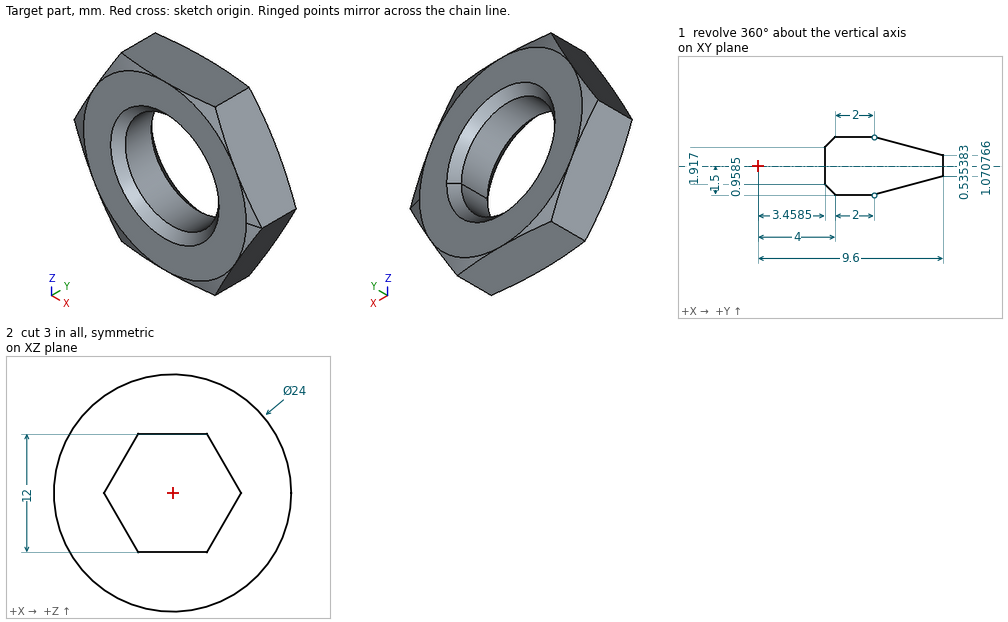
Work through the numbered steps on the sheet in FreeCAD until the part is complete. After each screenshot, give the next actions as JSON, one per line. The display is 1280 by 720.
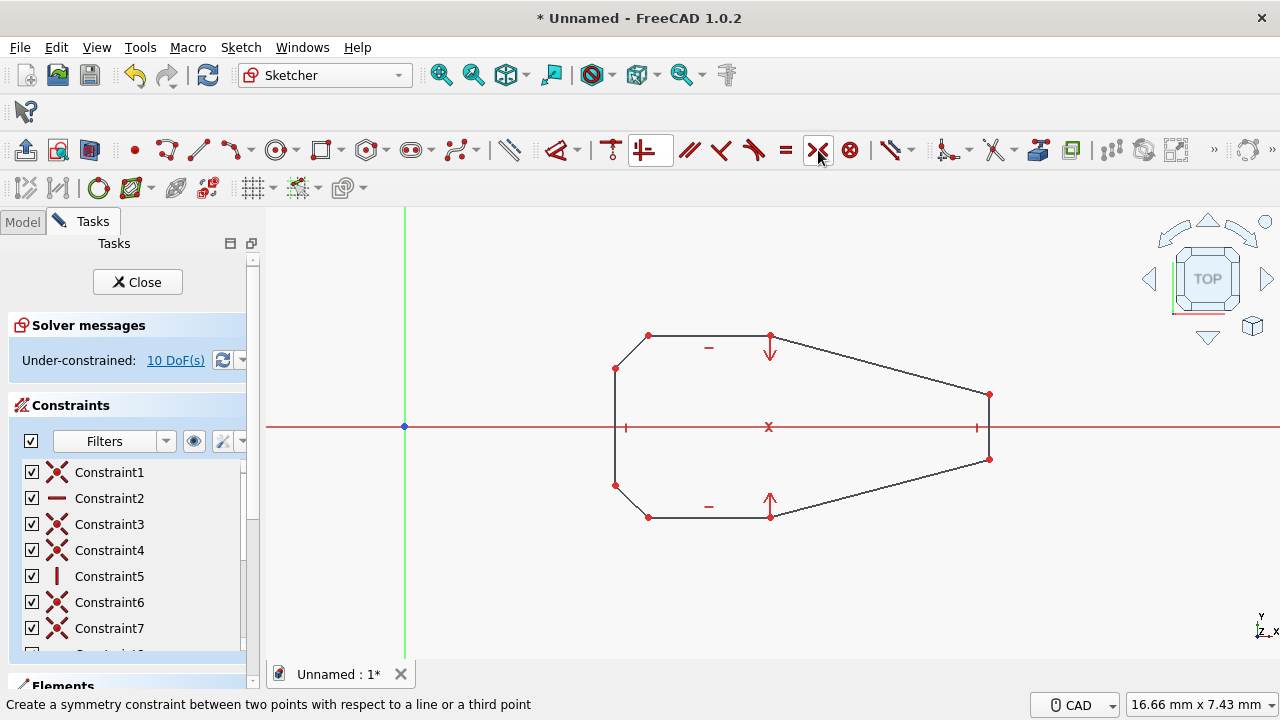
{"action": "left_click", "coordinate": [556, 150]}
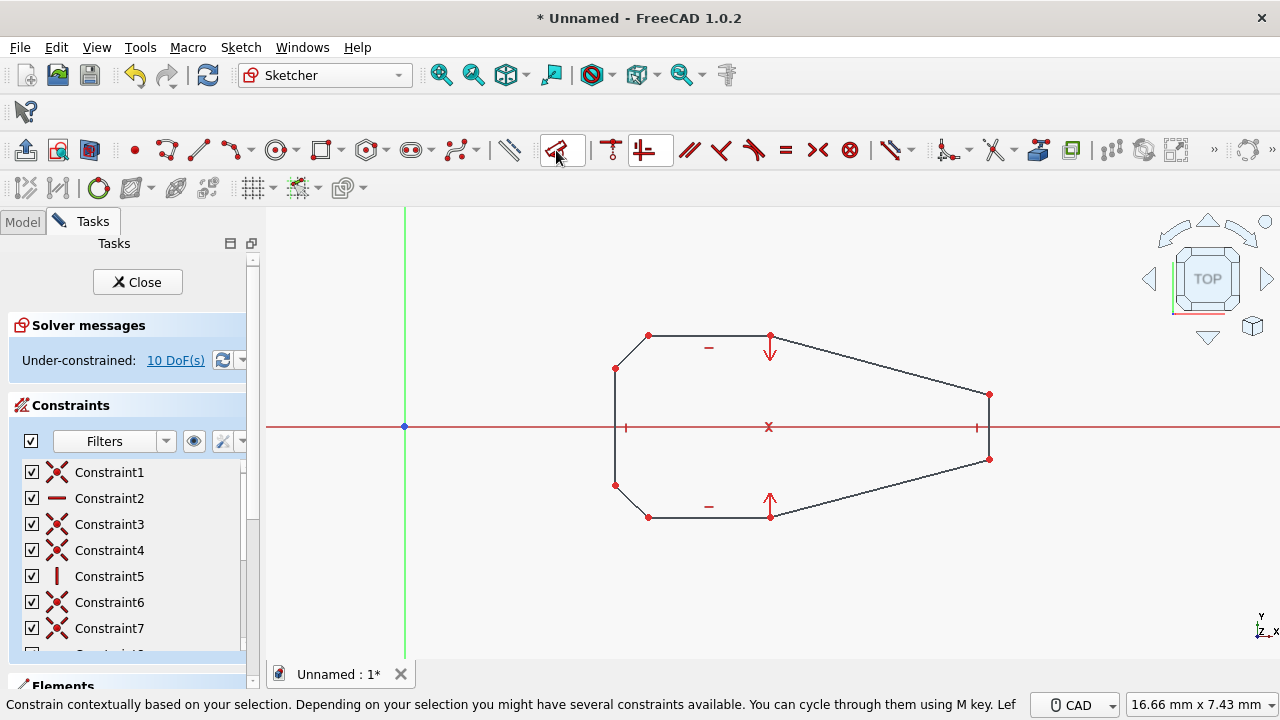
{"action": "left_click", "coordinate": [685, 518]}
{"action": "left_click", "coordinate": [709, 552]}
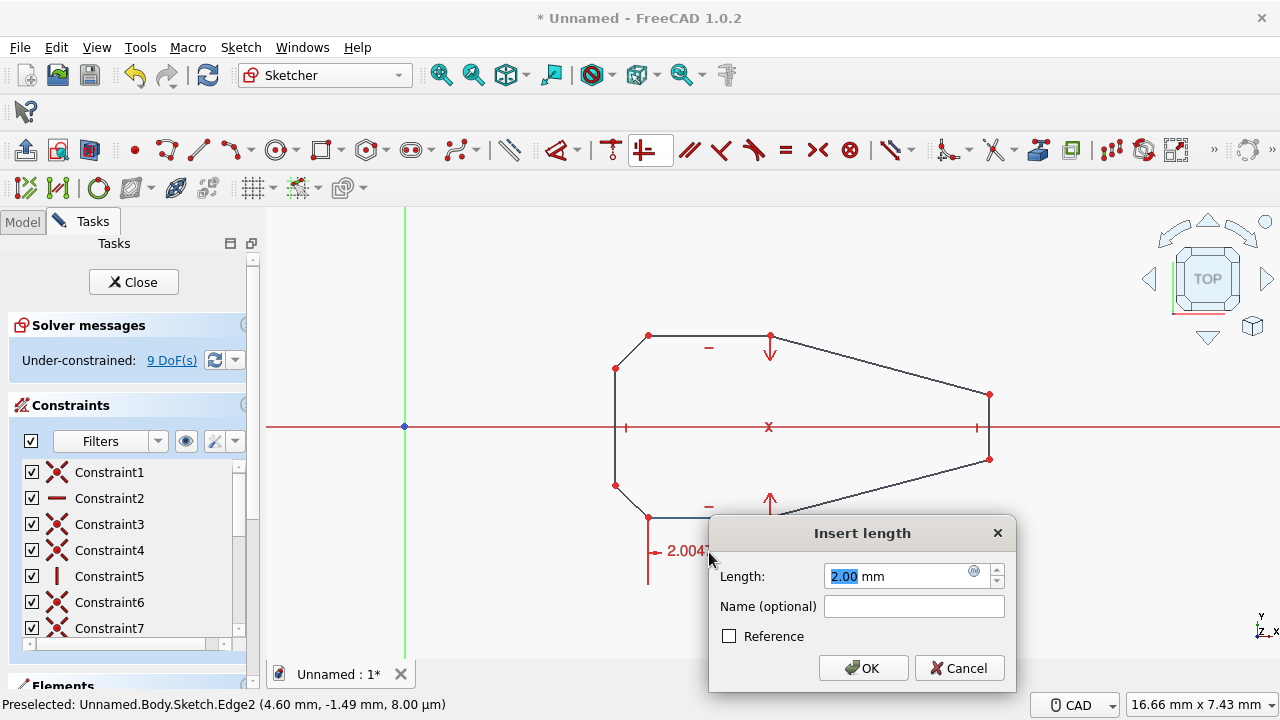
{"action": "type", "text": "2"}
{"action": "key", "text": "Return"}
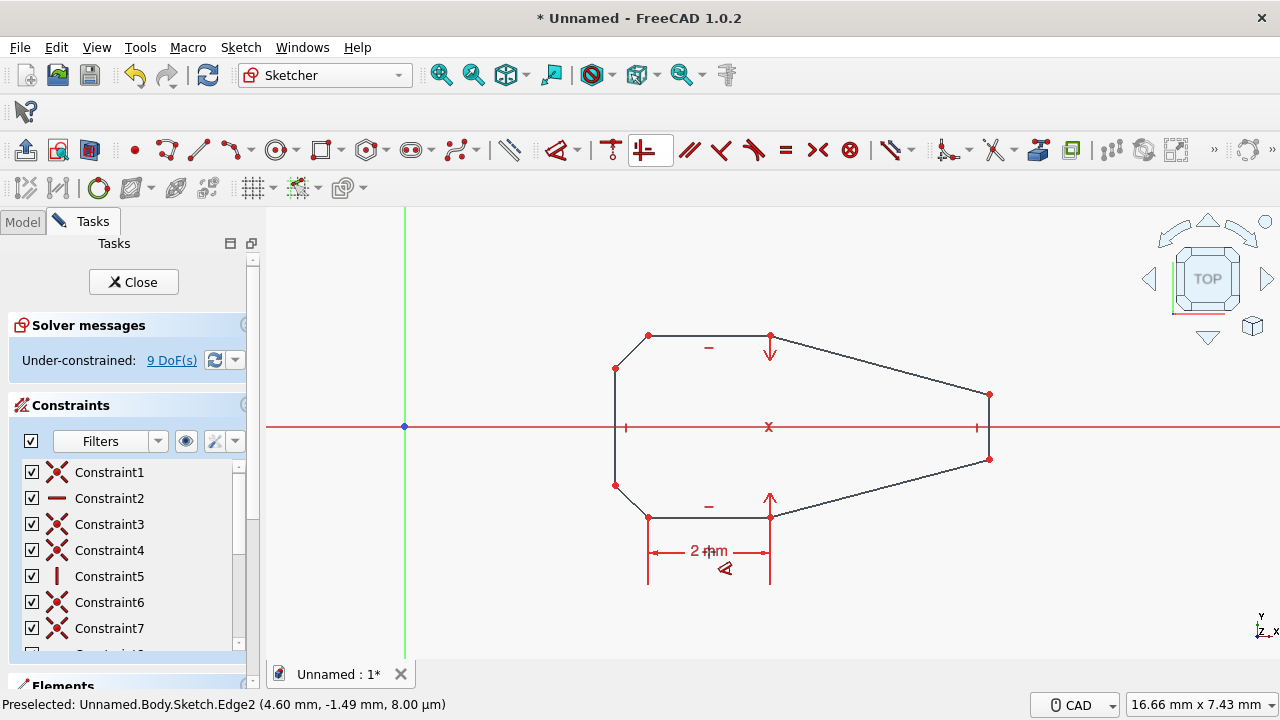
{"action": "left_click", "coordinate": [733, 336]}
{"action": "left_click", "coordinate": [709, 302]}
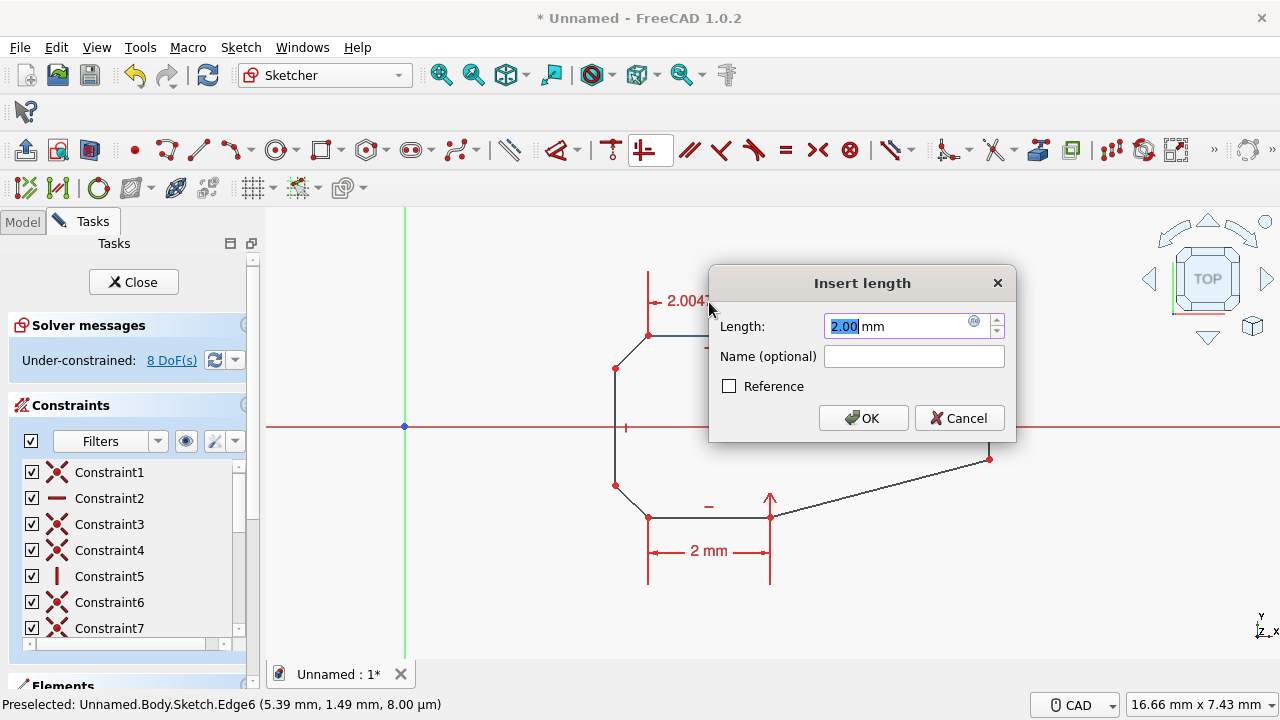
{"action": "type", "text": "2"}
{"action": "key", "text": "Return"}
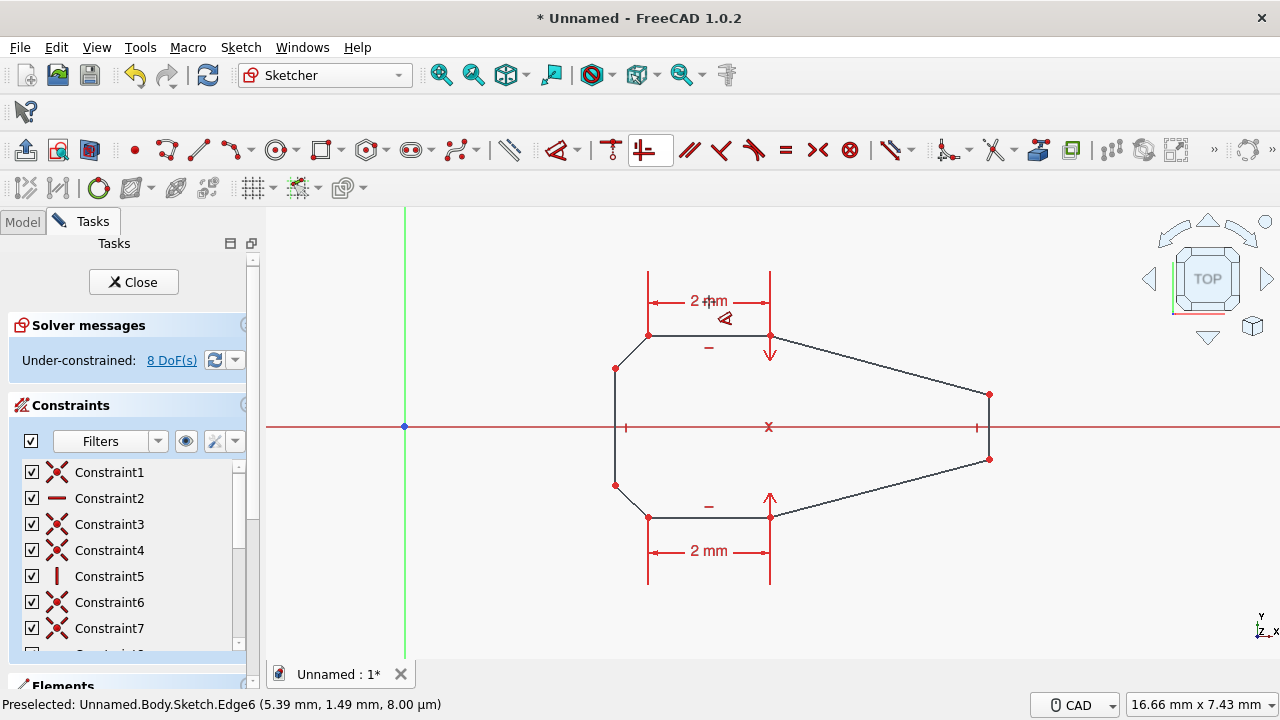
{"action": "left_click", "coordinate": [648, 518]}
{"action": "left_click", "coordinate": [527, 552]}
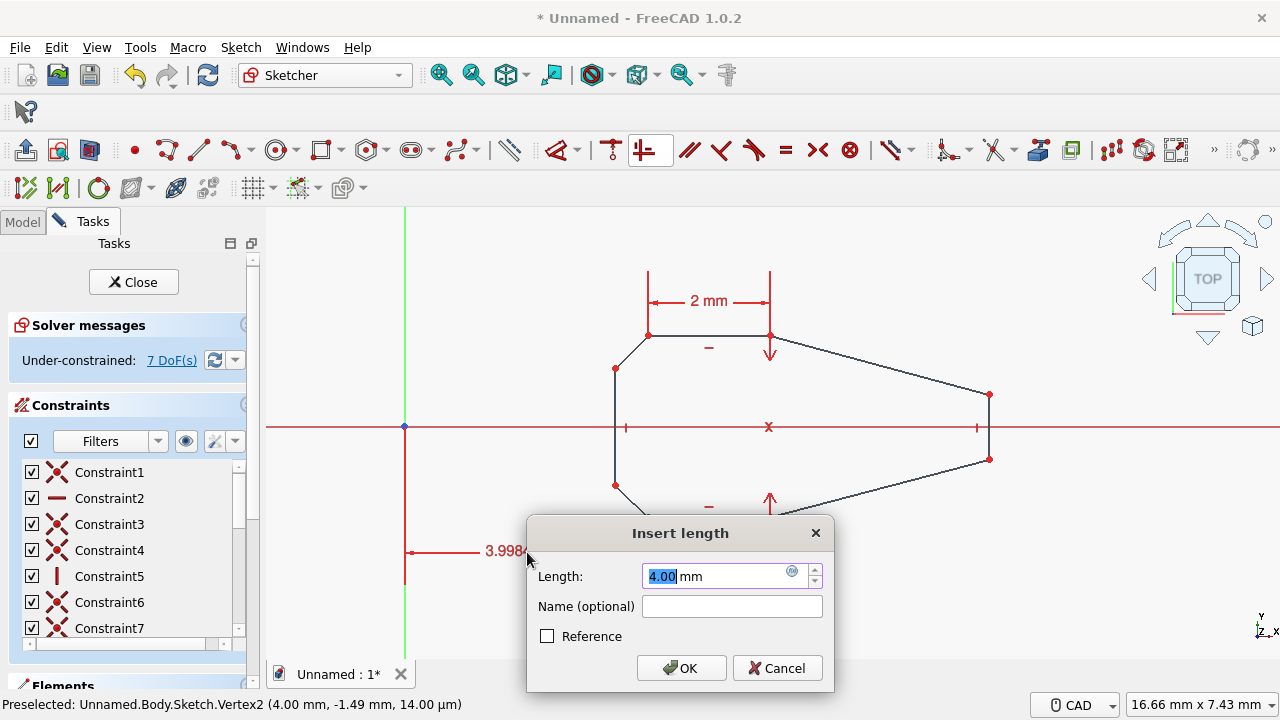
{"action": "type", "text": "4"}
{"action": "key", "text": "Return"}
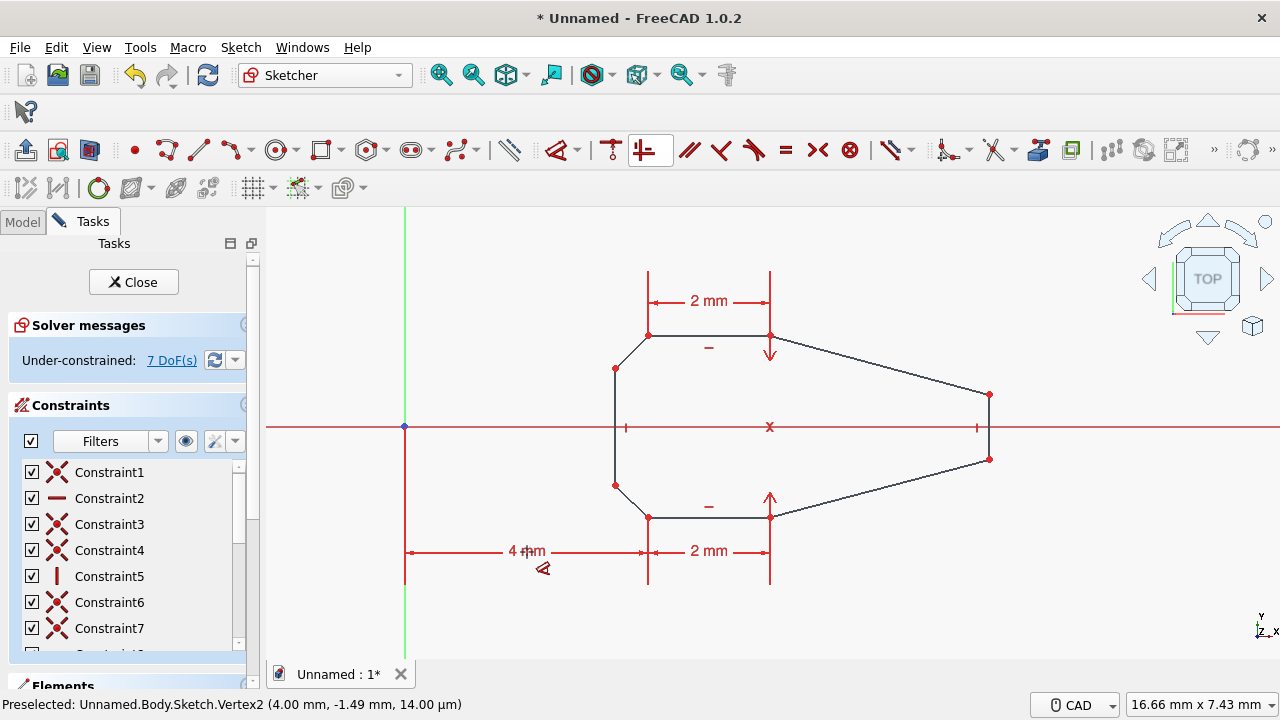
{"action": "left_click", "coordinate": [648, 518]}
{"action": "left_click", "coordinate": [371, 472]}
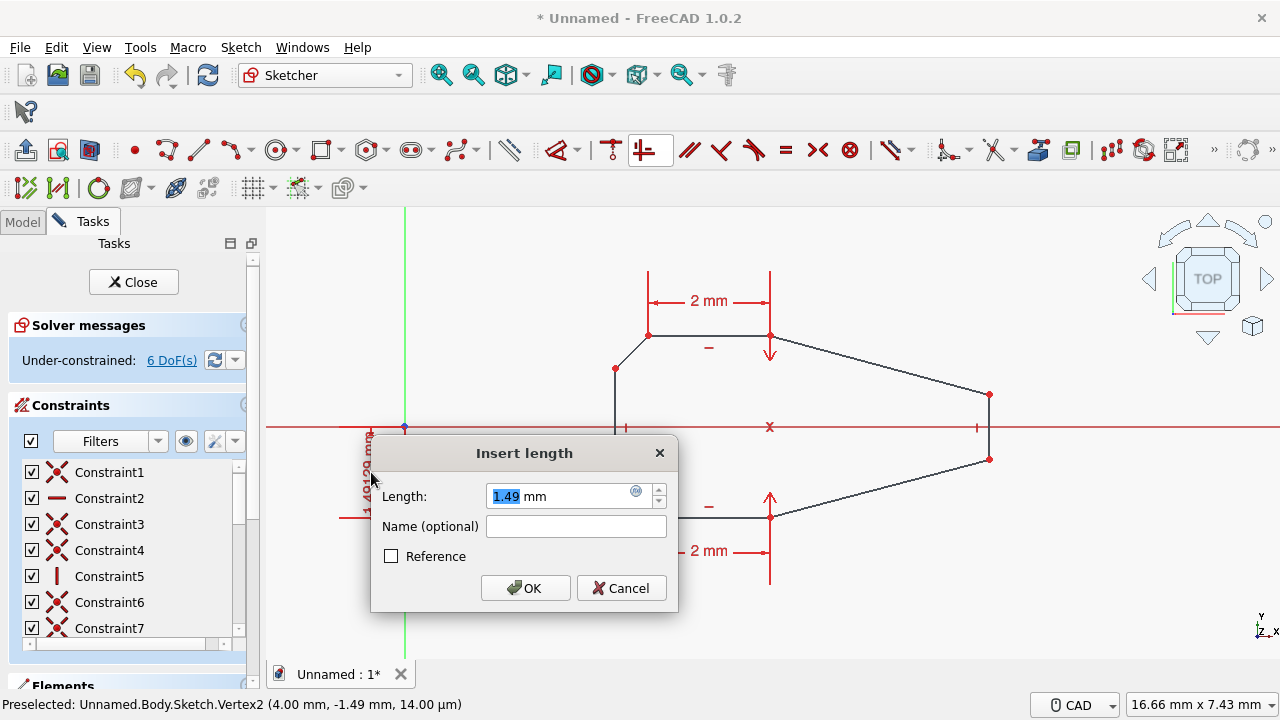
{"action": "type", "text": "1.5"}
{"action": "key", "text": "Return"}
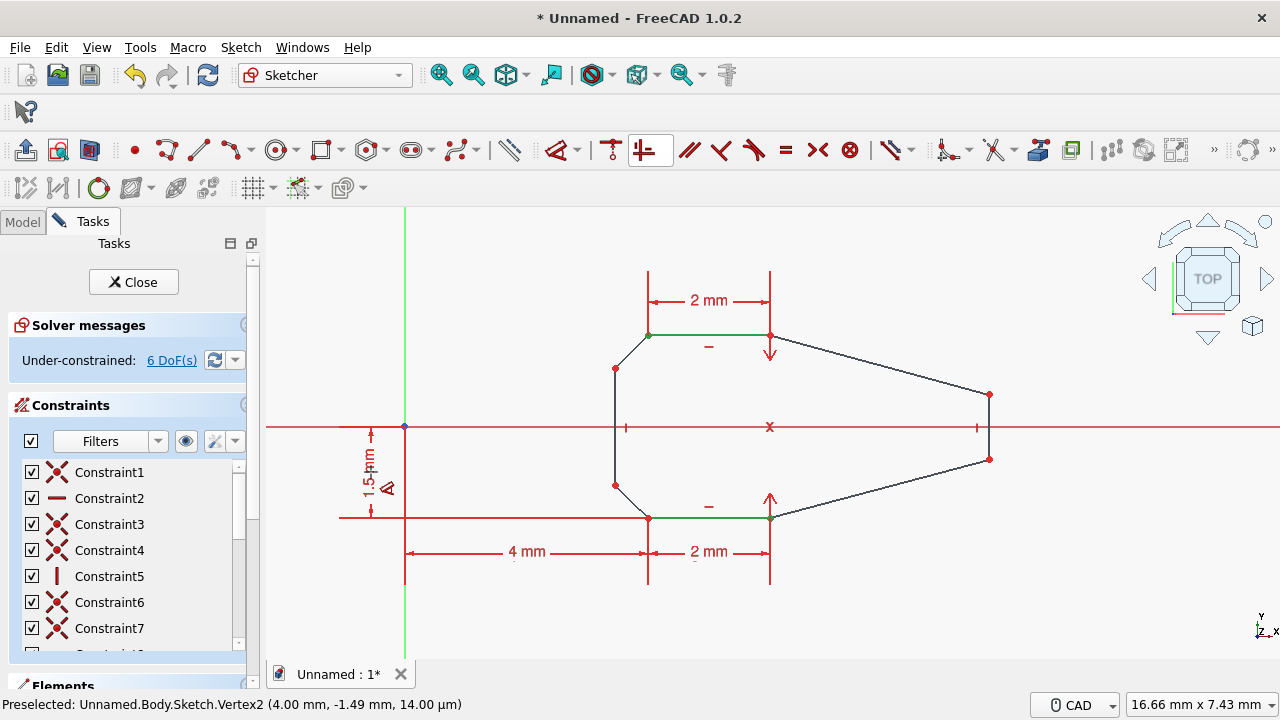
{"action": "left_click", "coordinate": [989, 460]}
{"action": "left_click", "coordinate": [697, 494]}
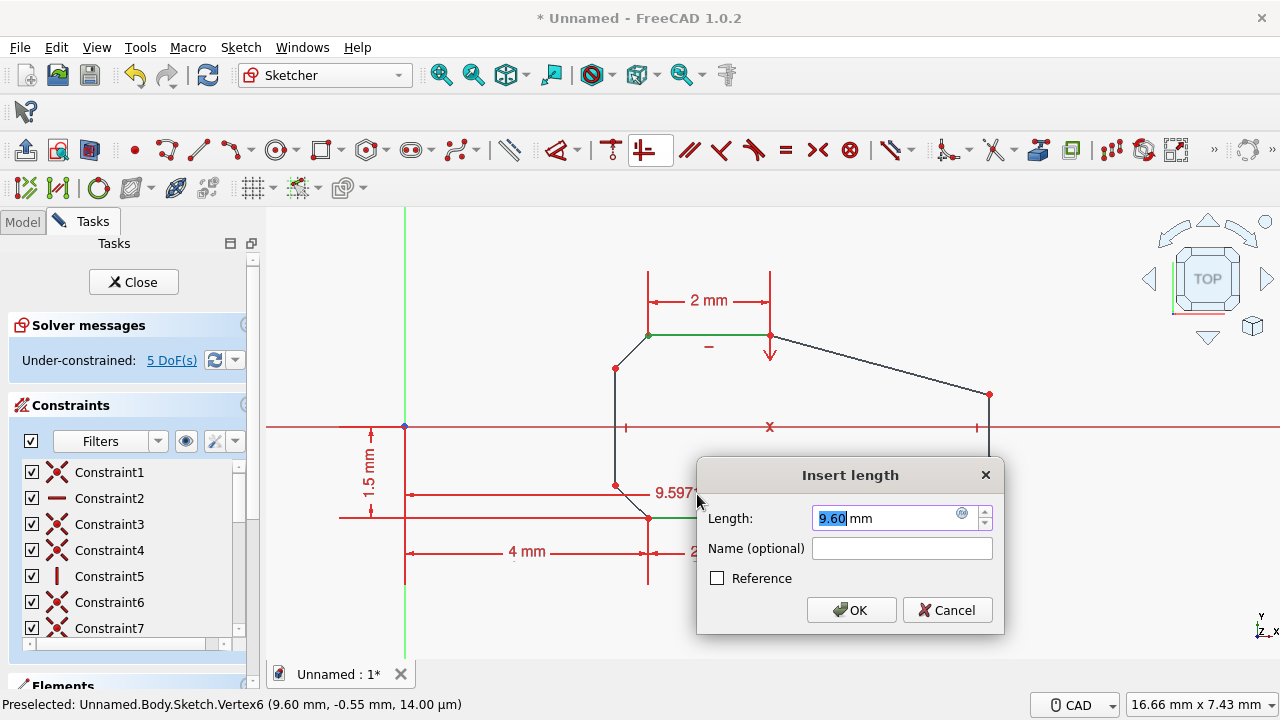
{"action": "type", "text": "9.6"}
{"action": "key", "text": "Return"}